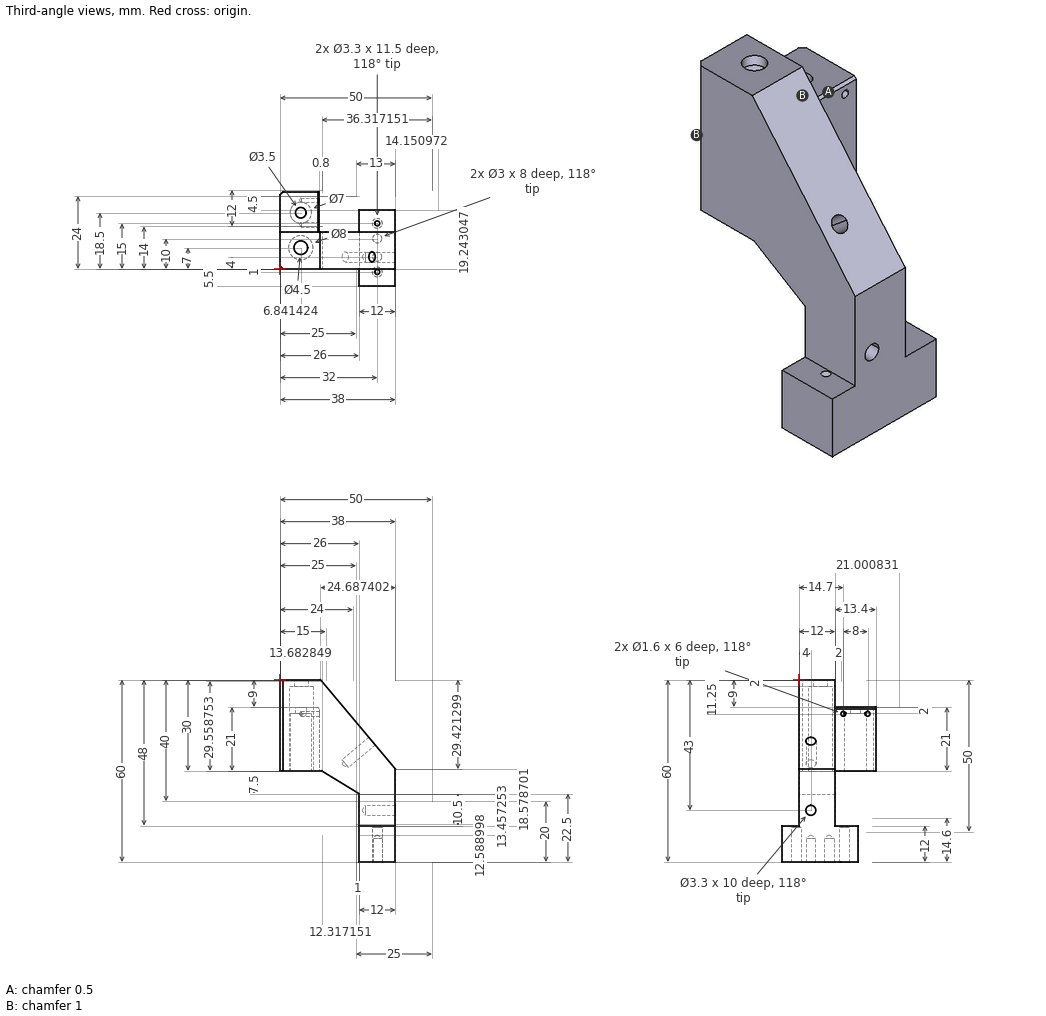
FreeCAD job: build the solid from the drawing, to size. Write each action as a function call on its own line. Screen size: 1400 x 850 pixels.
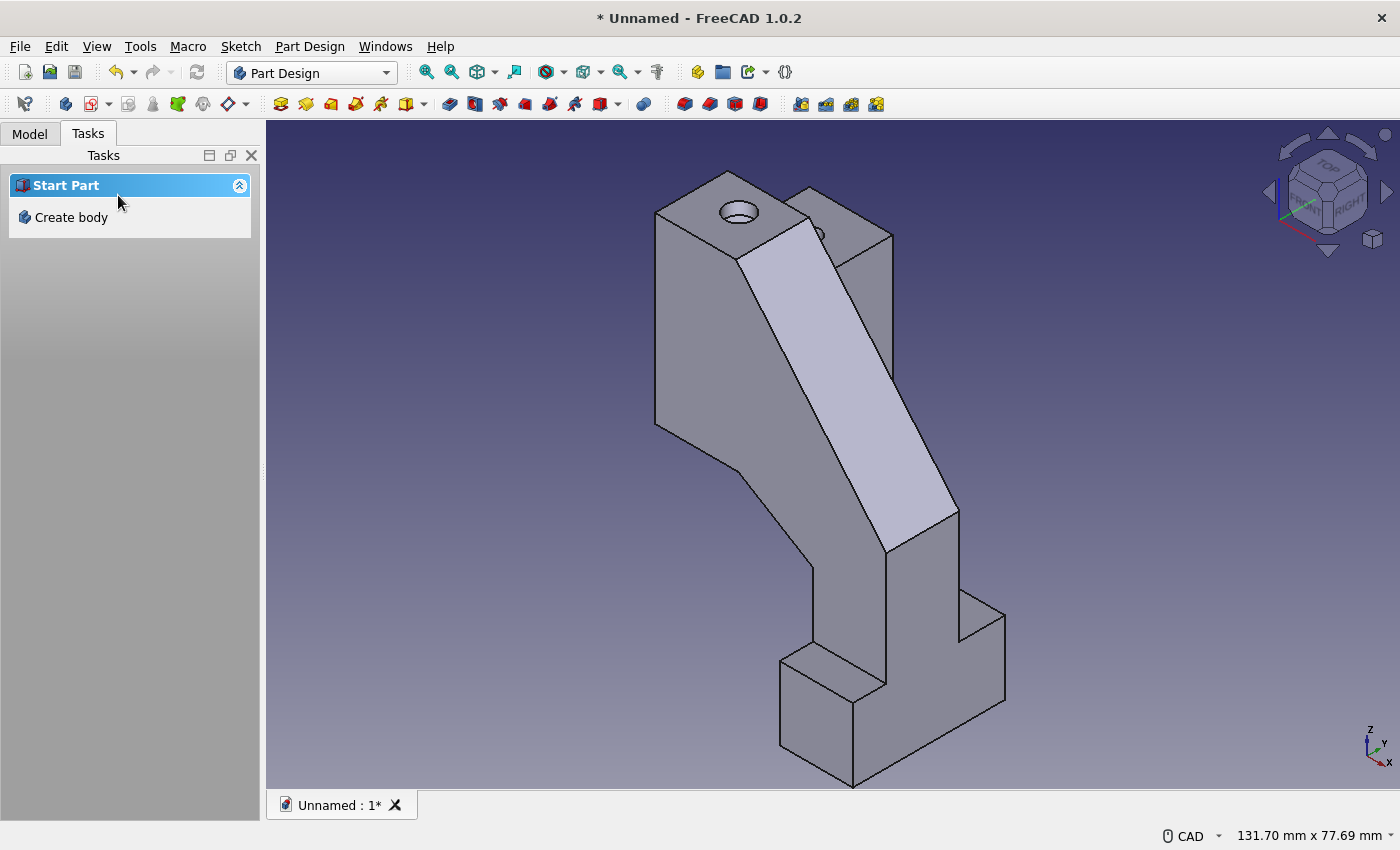
key(3)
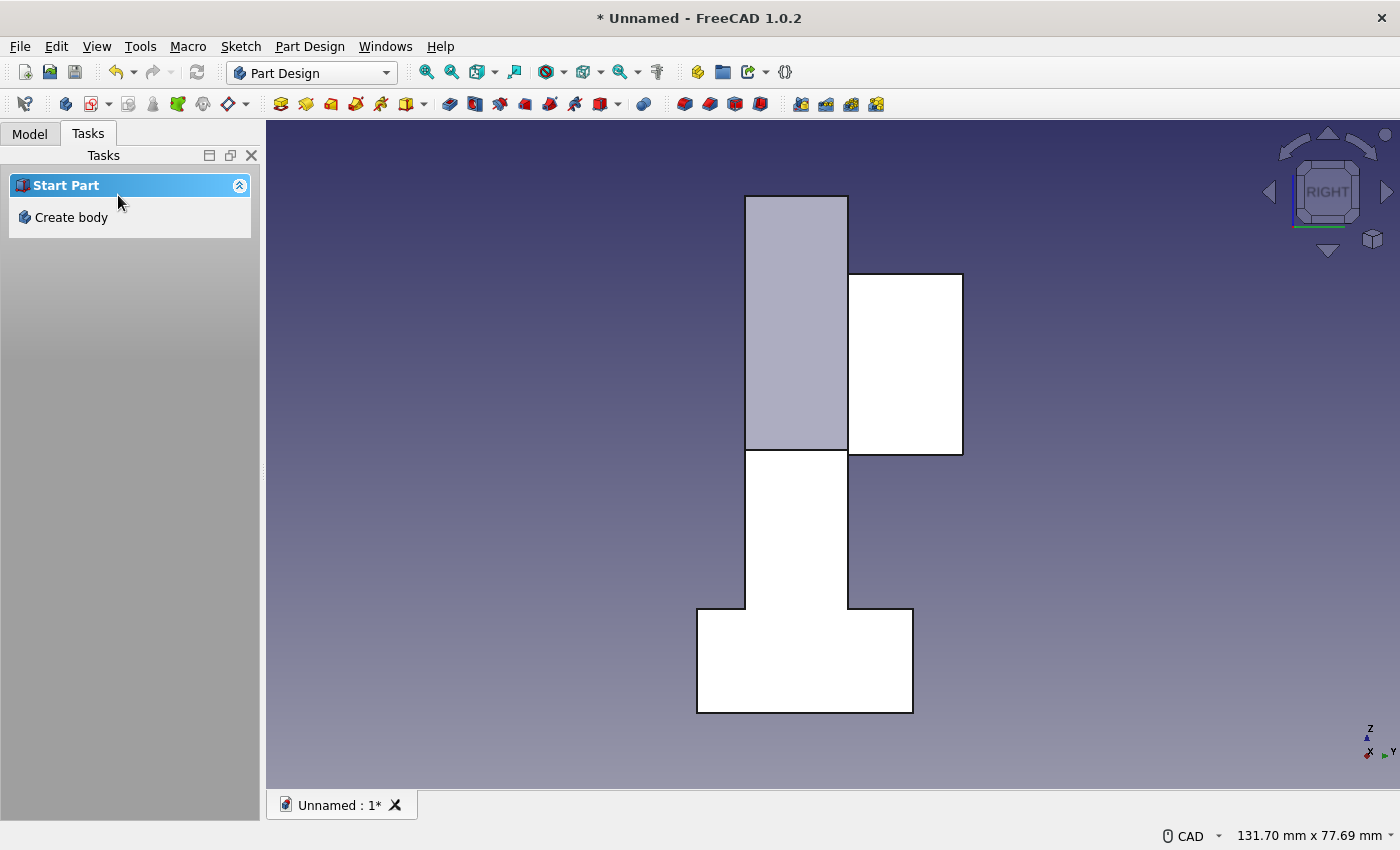
click(906, 363)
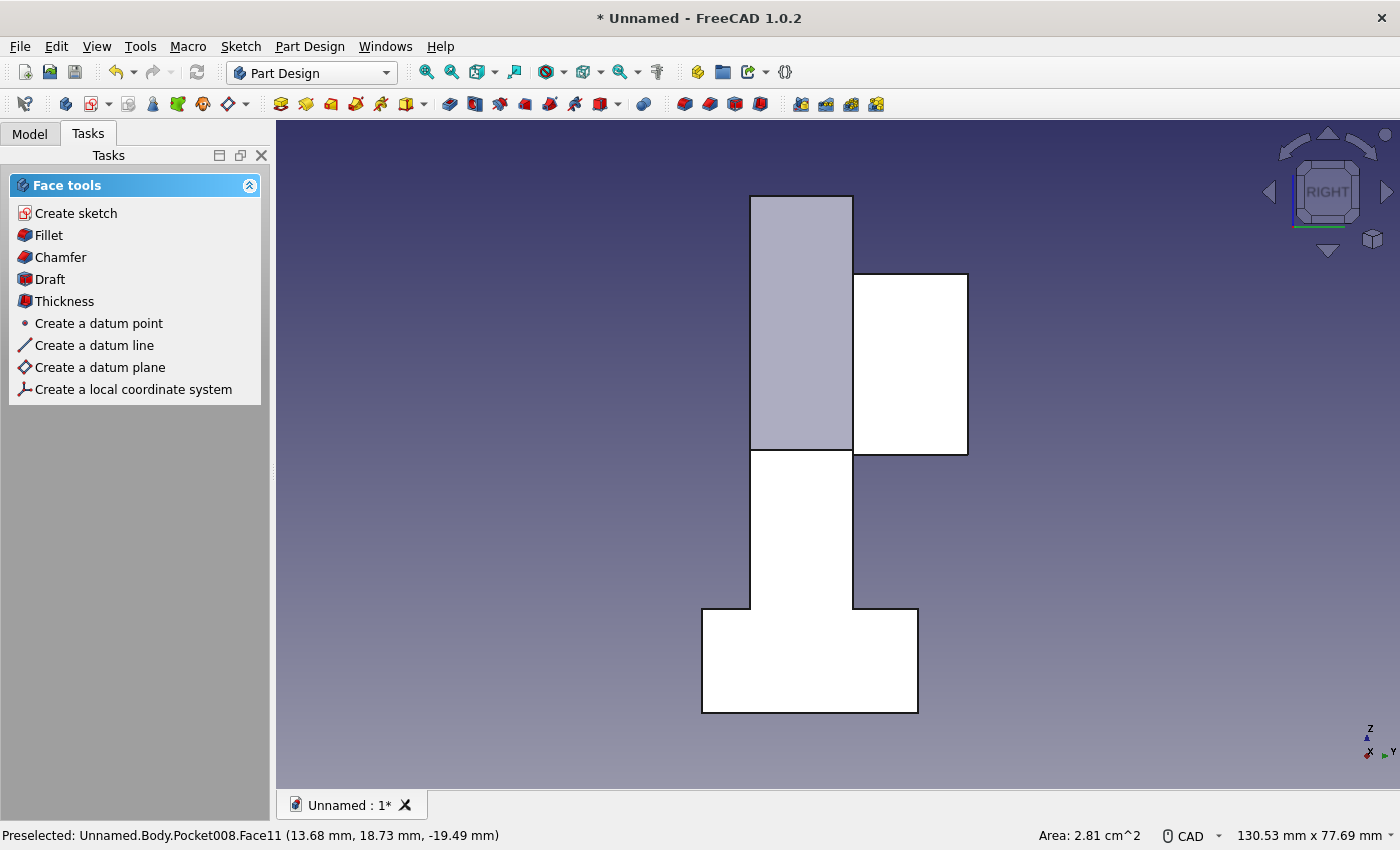
click(90, 104)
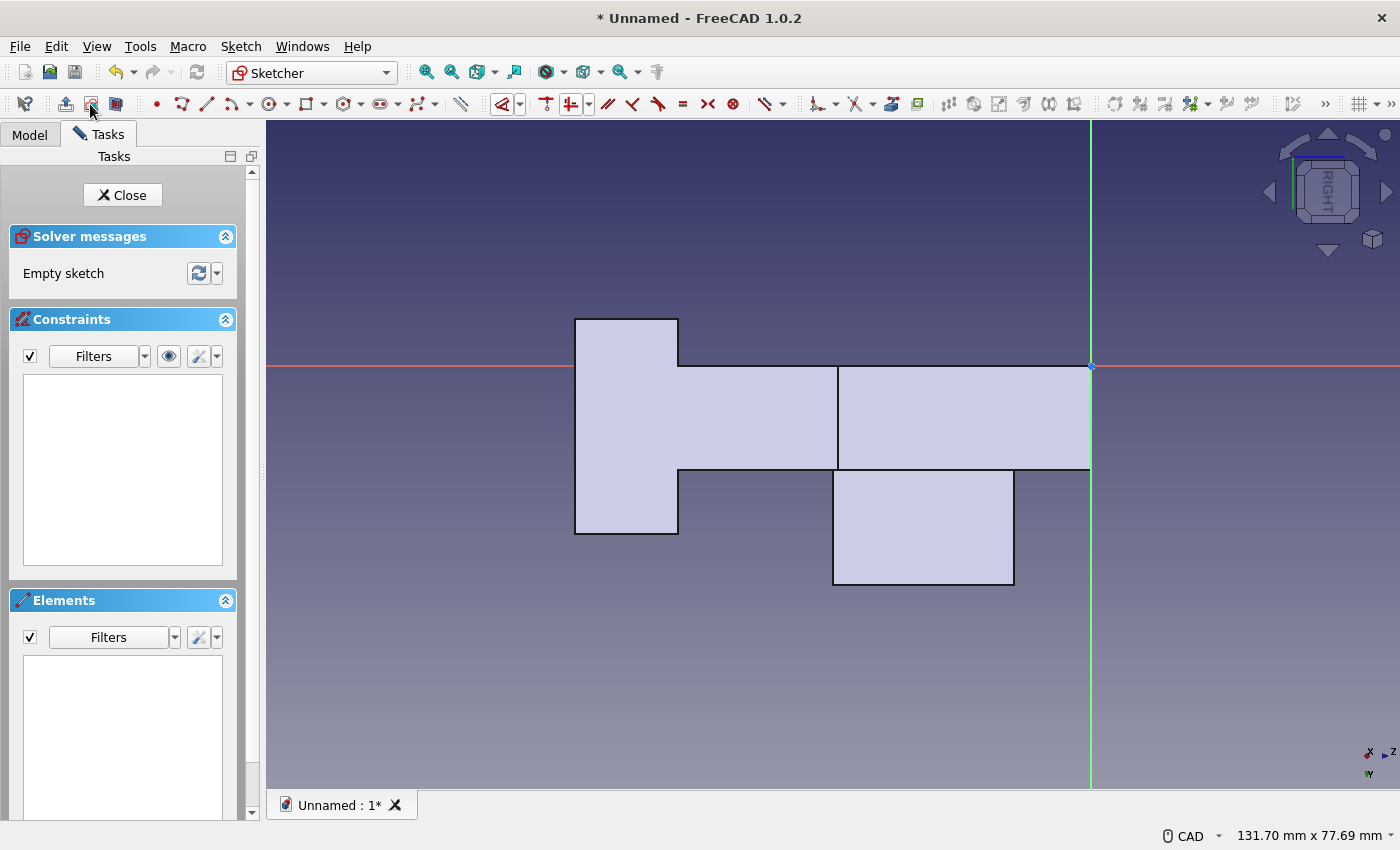
click(116, 104)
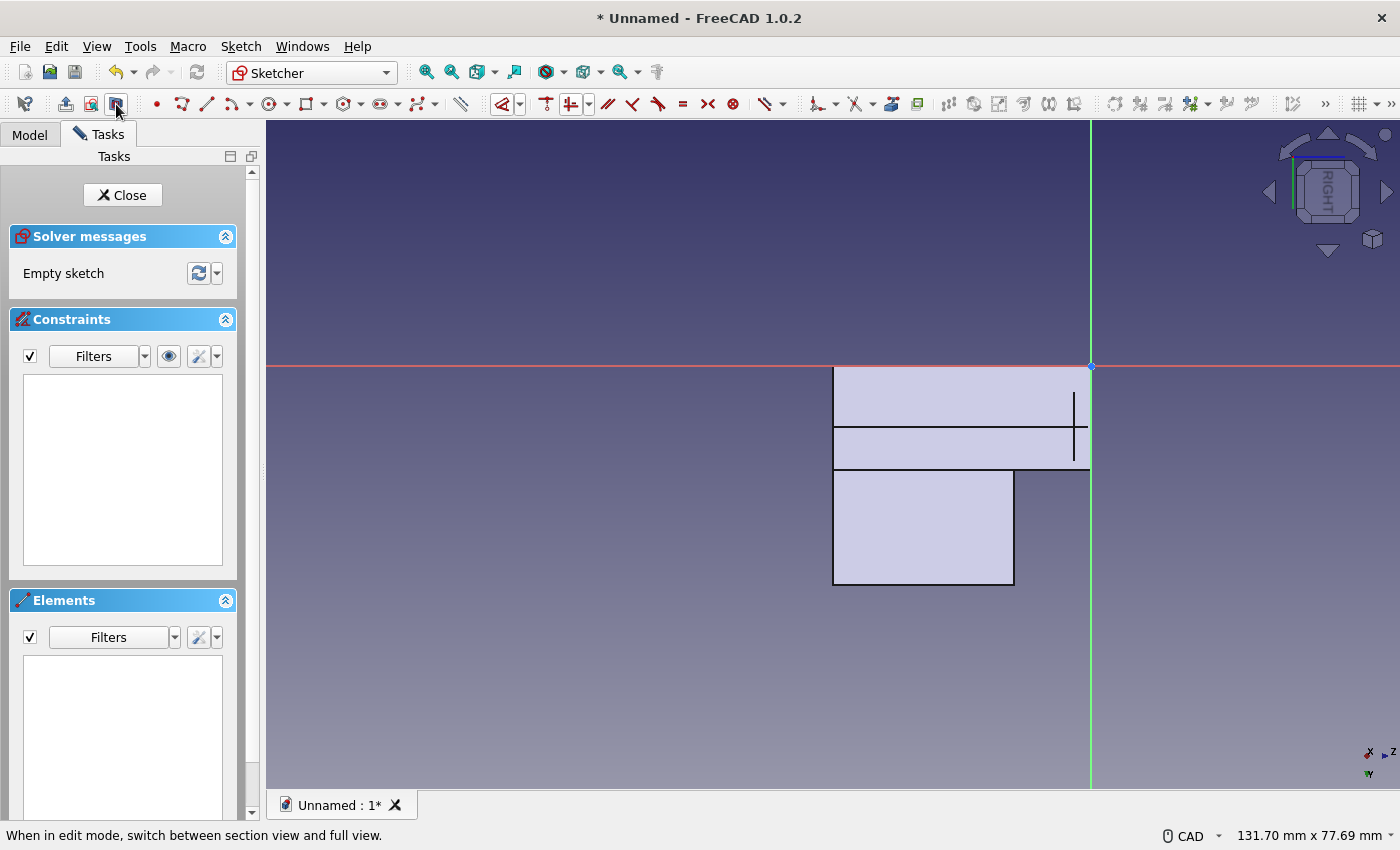
scroll(1203, 501, up, 3)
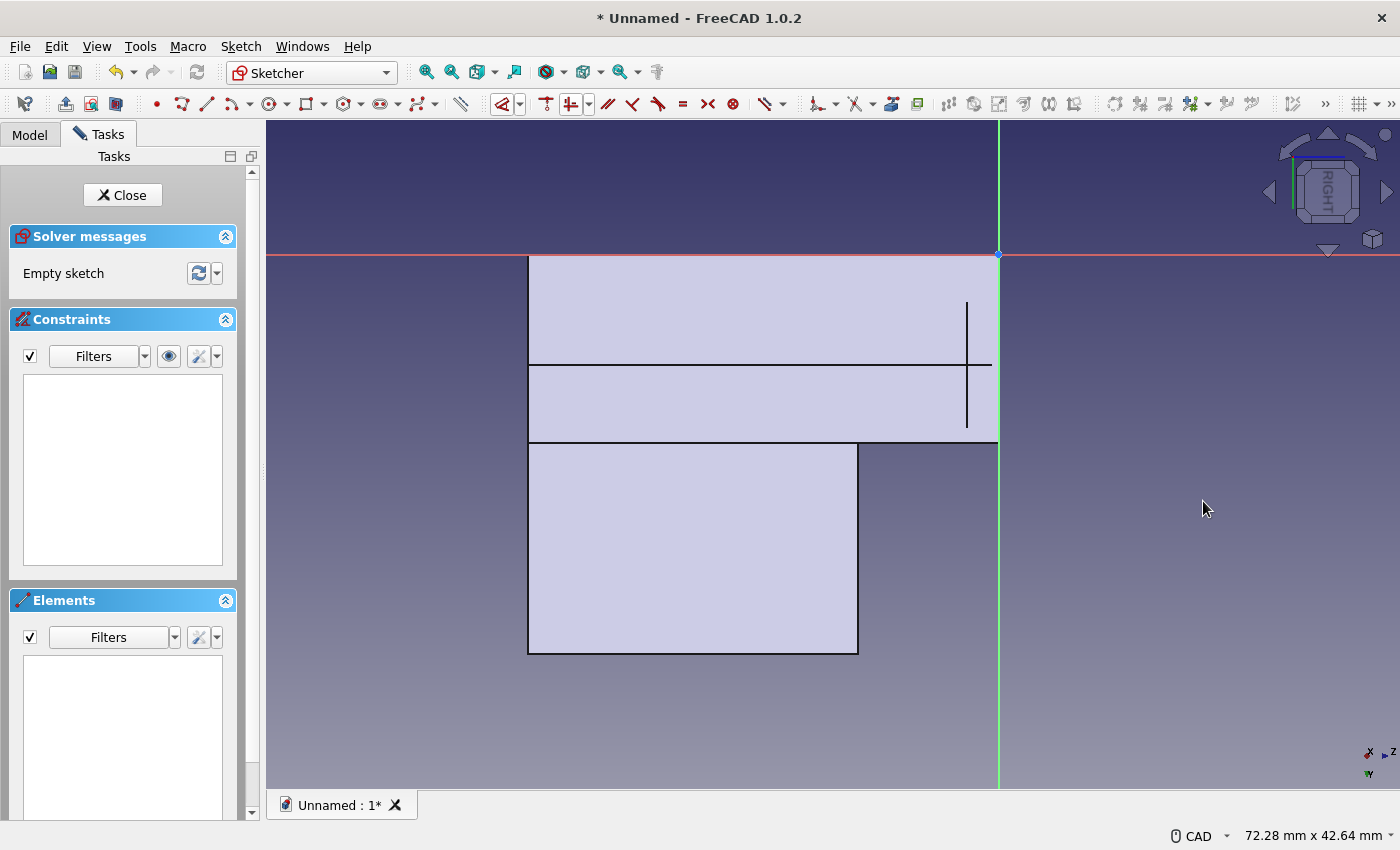
key(g)
key(r)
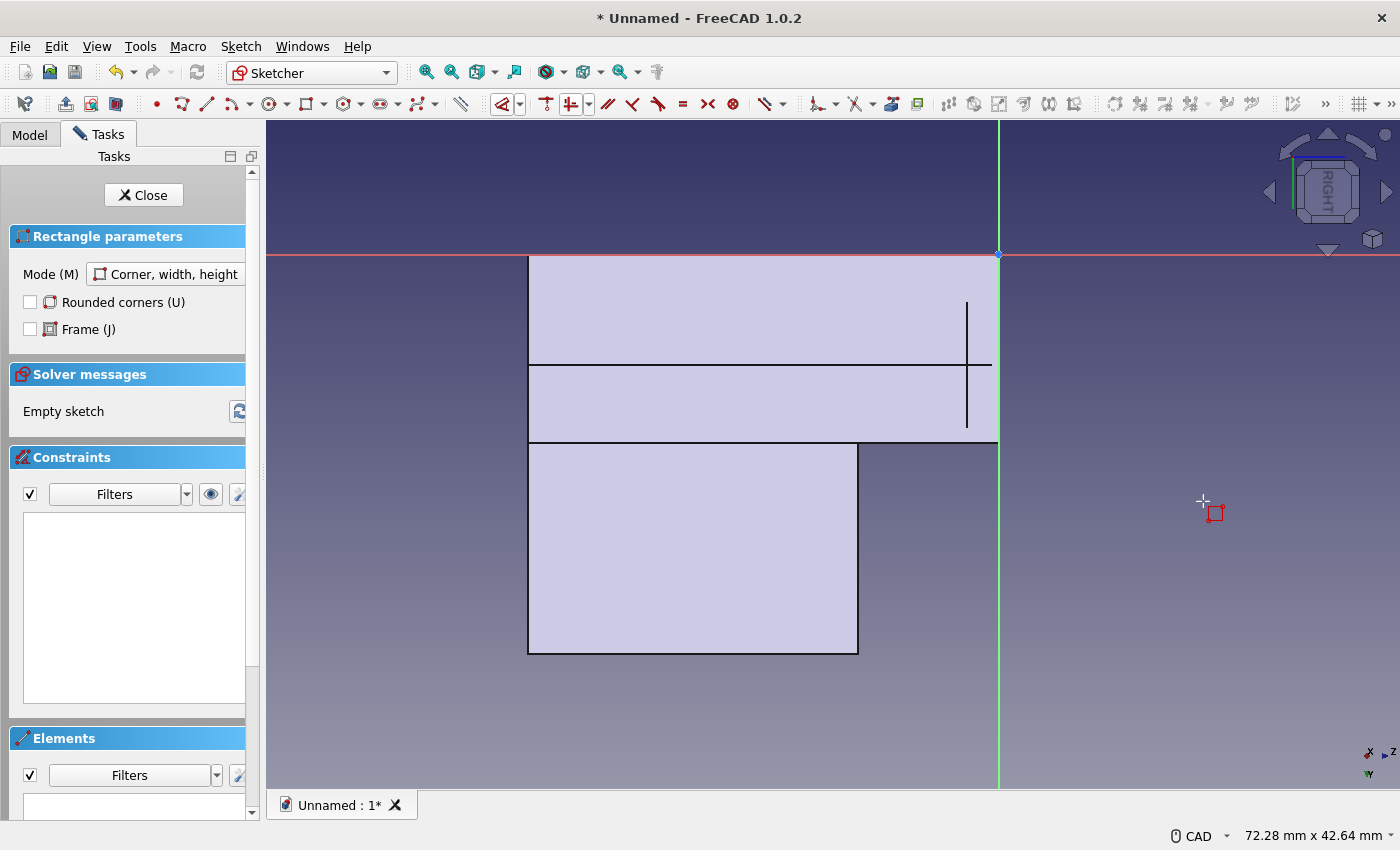
click(528, 443)
click(858, 654)
key(Escape)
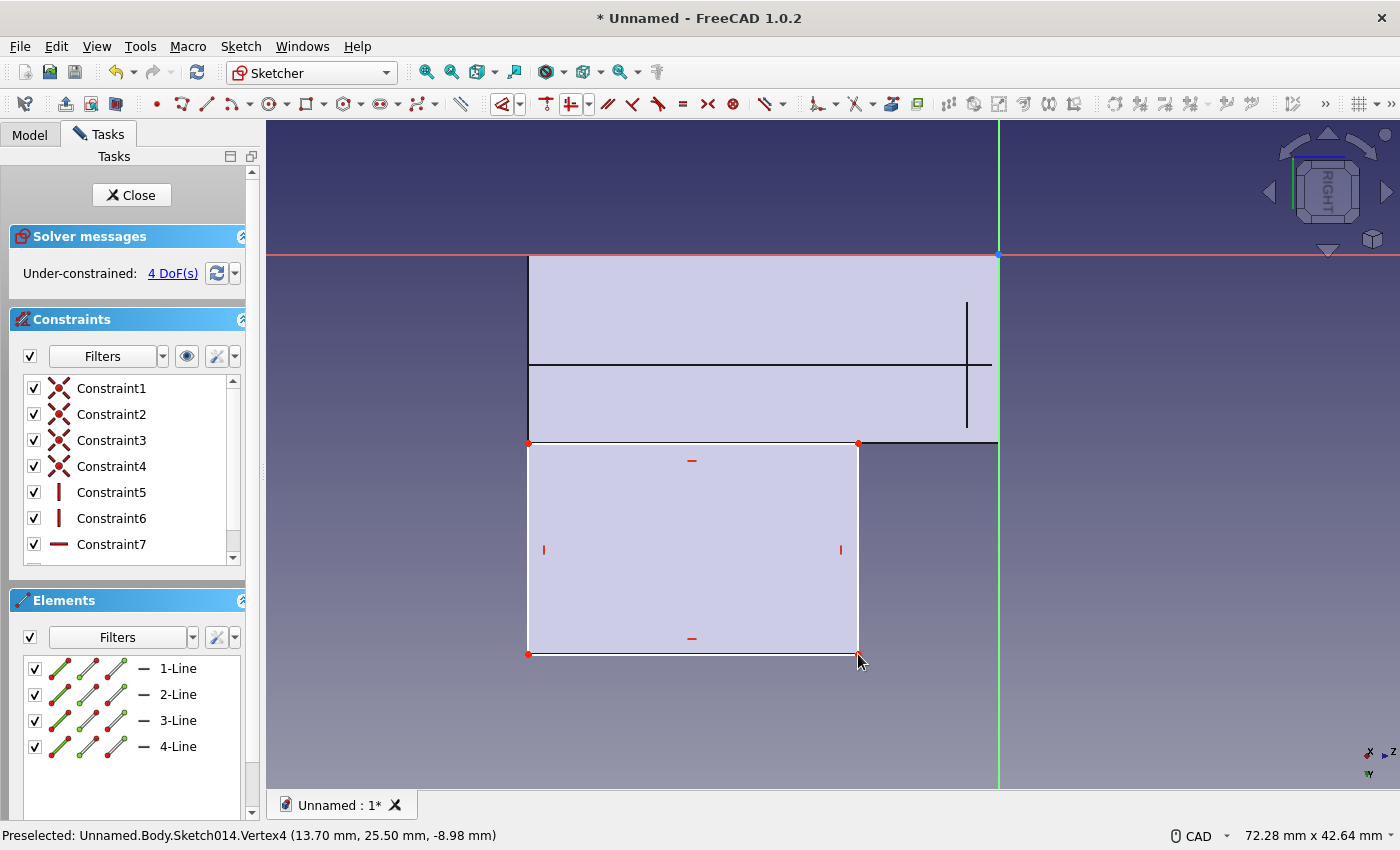
click(627, 655)